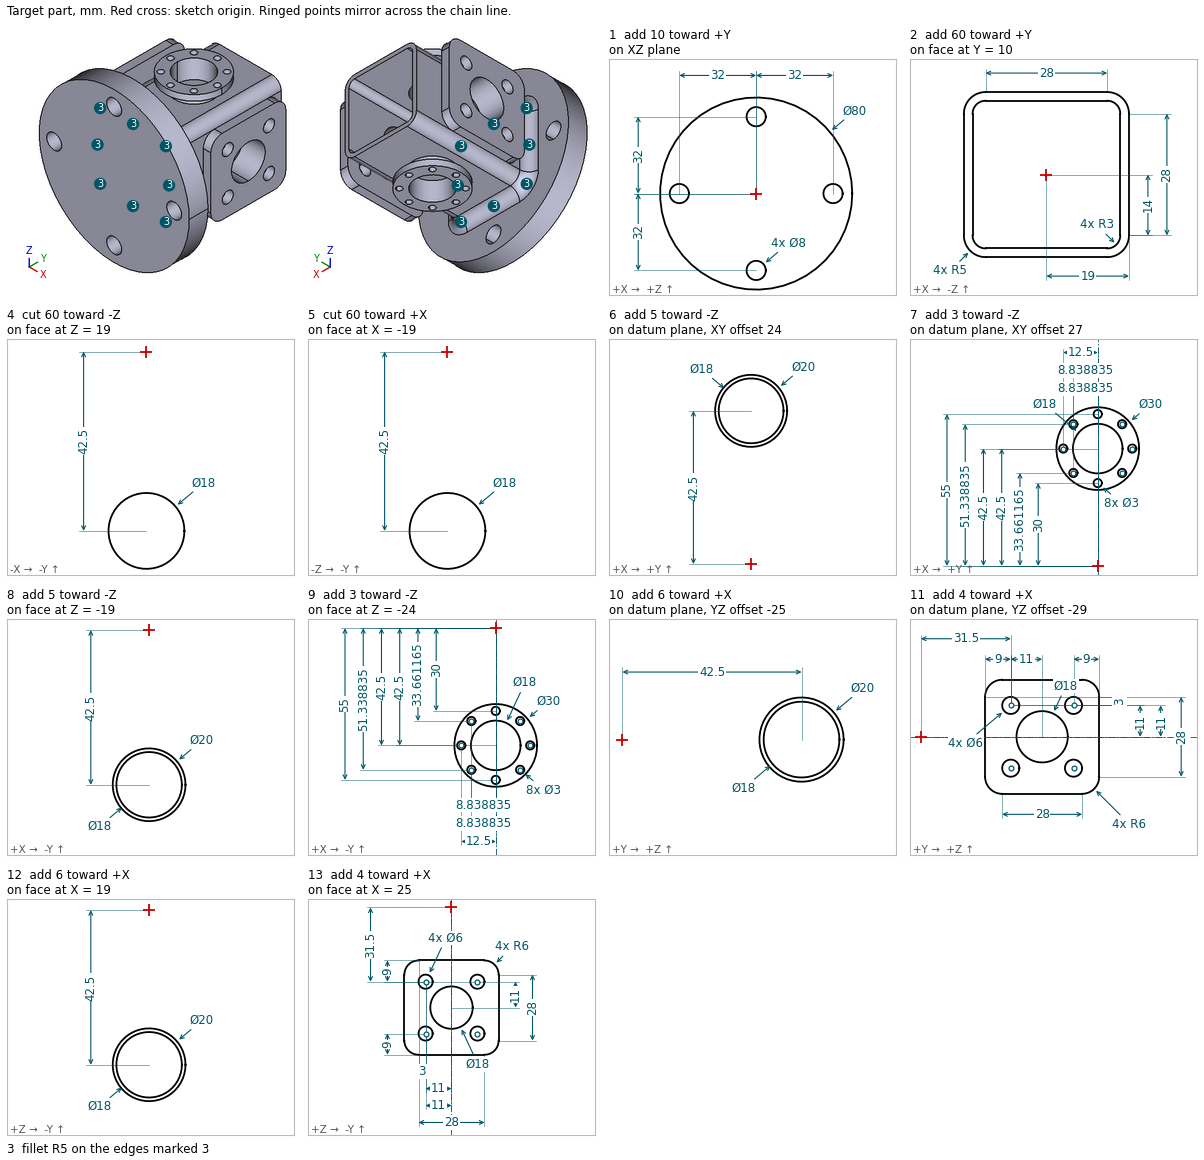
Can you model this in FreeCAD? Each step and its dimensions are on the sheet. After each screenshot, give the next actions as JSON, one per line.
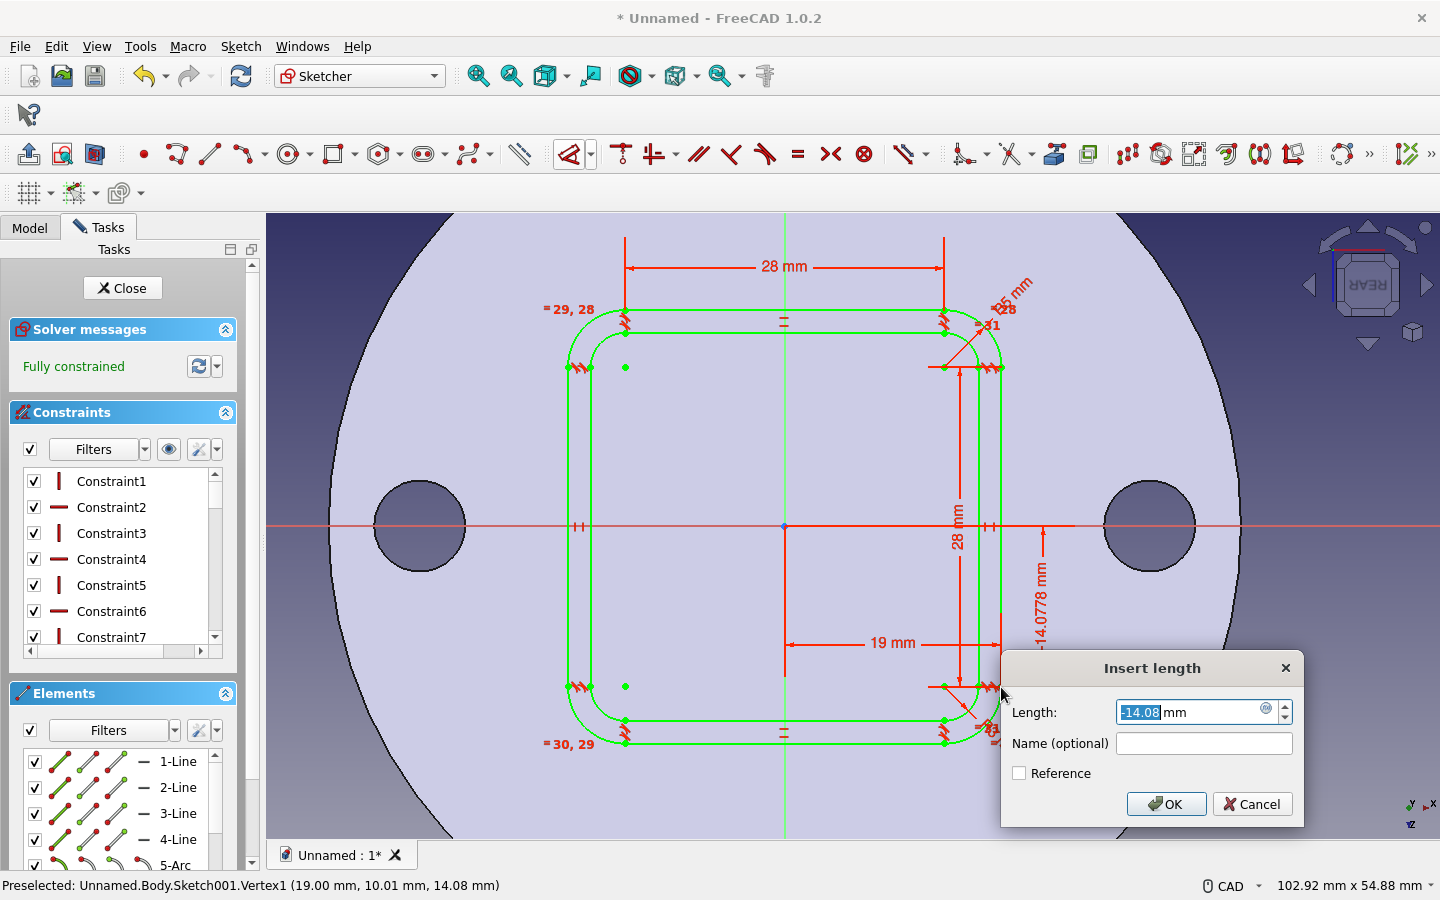
{"action": "type", "text": "-14"}
{"action": "key", "text": "Return"}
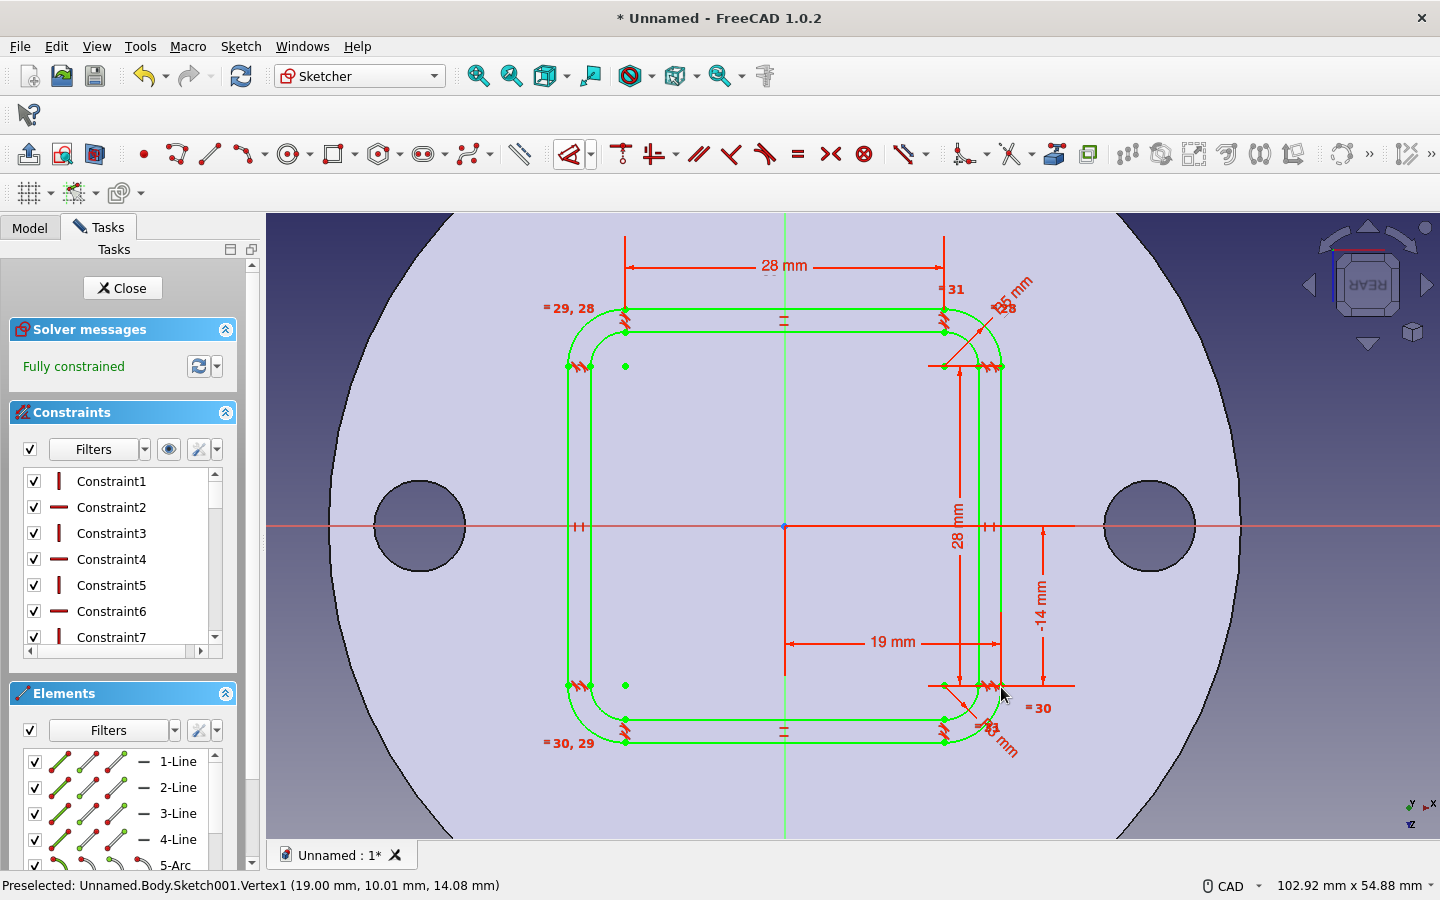
{"action": "left_click", "coordinate": [123, 288]}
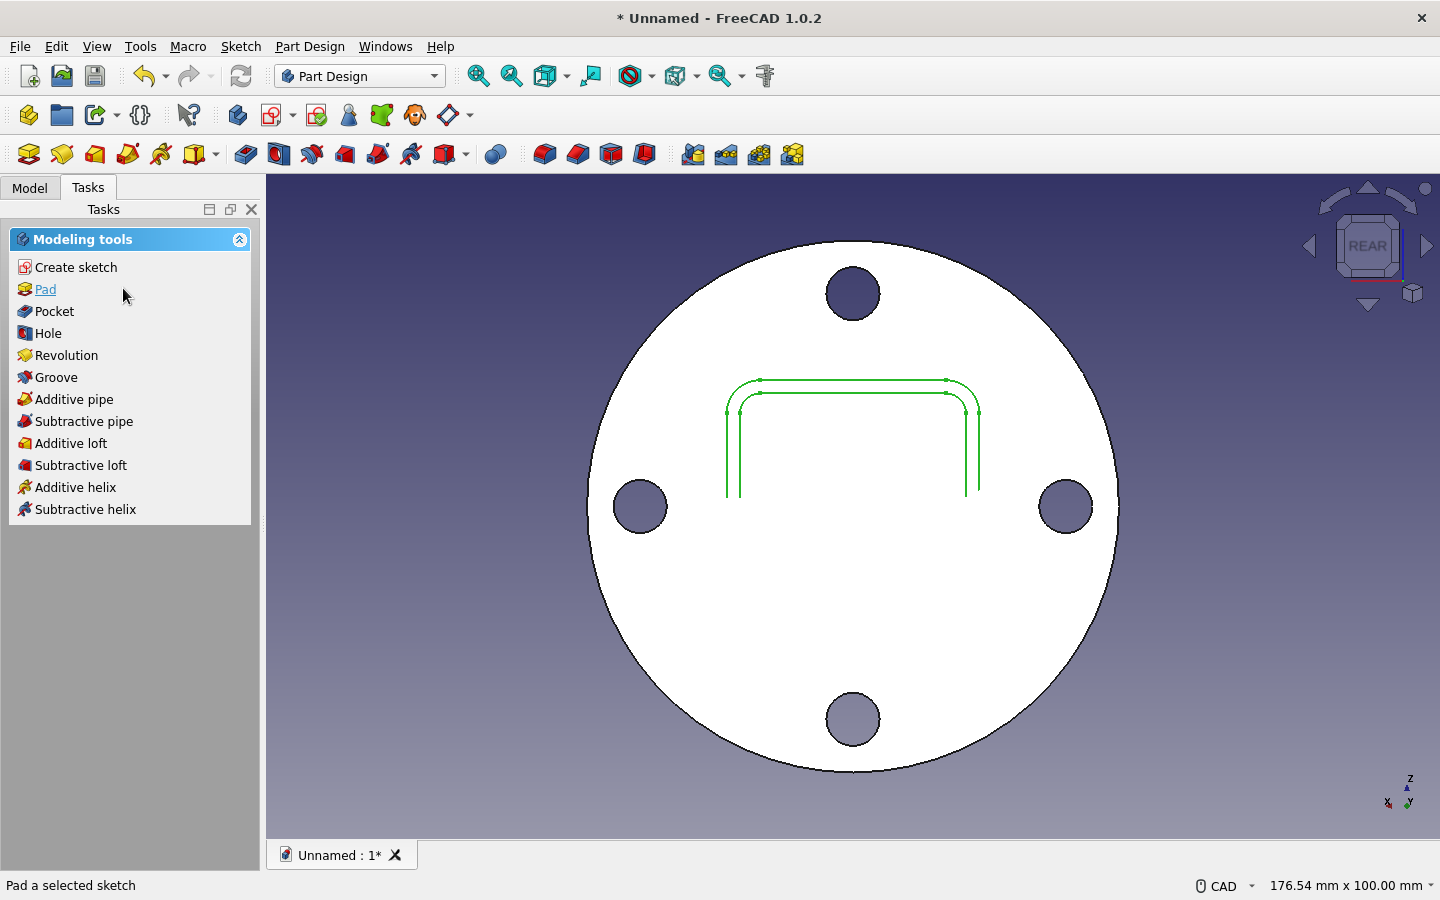
{"action": "left_click", "coordinate": [29, 154]}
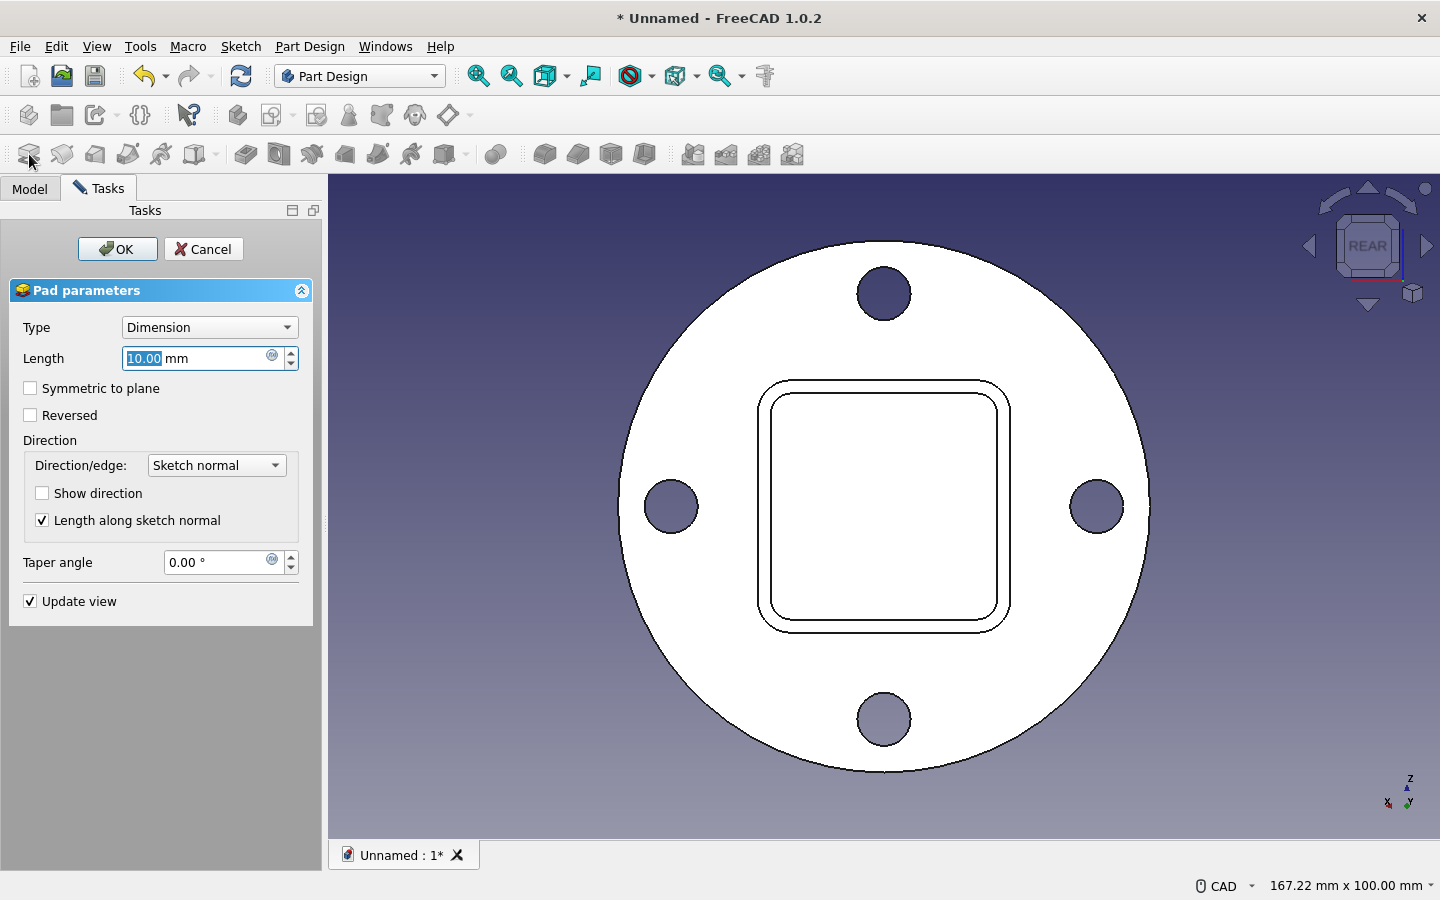
{"action": "type", "text": "60"}
{"action": "key", "text": "Tab"}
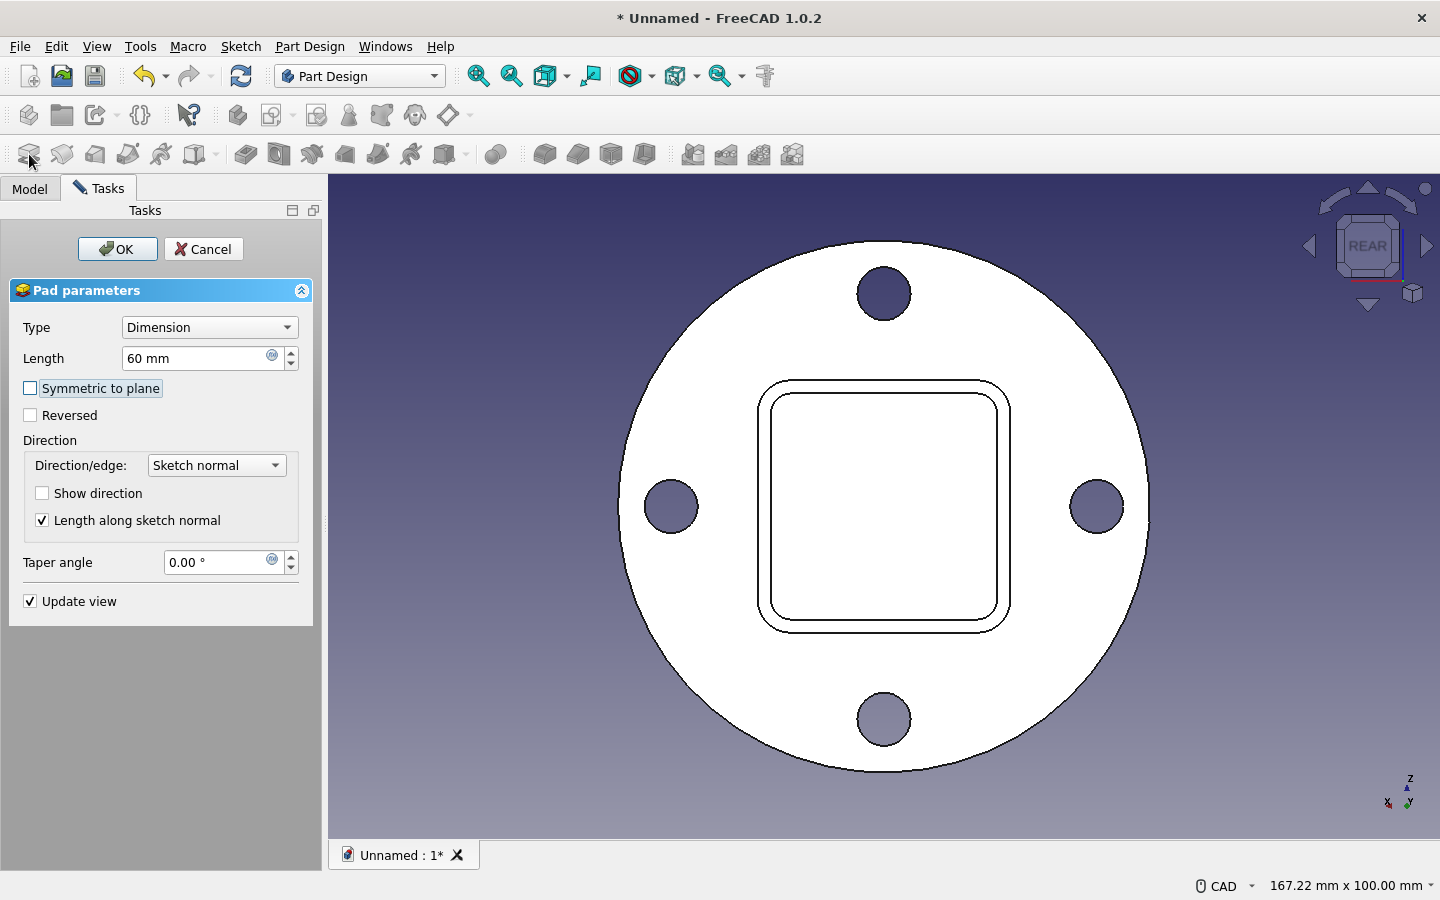
{"action": "left_click", "coordinate": [118, 249]}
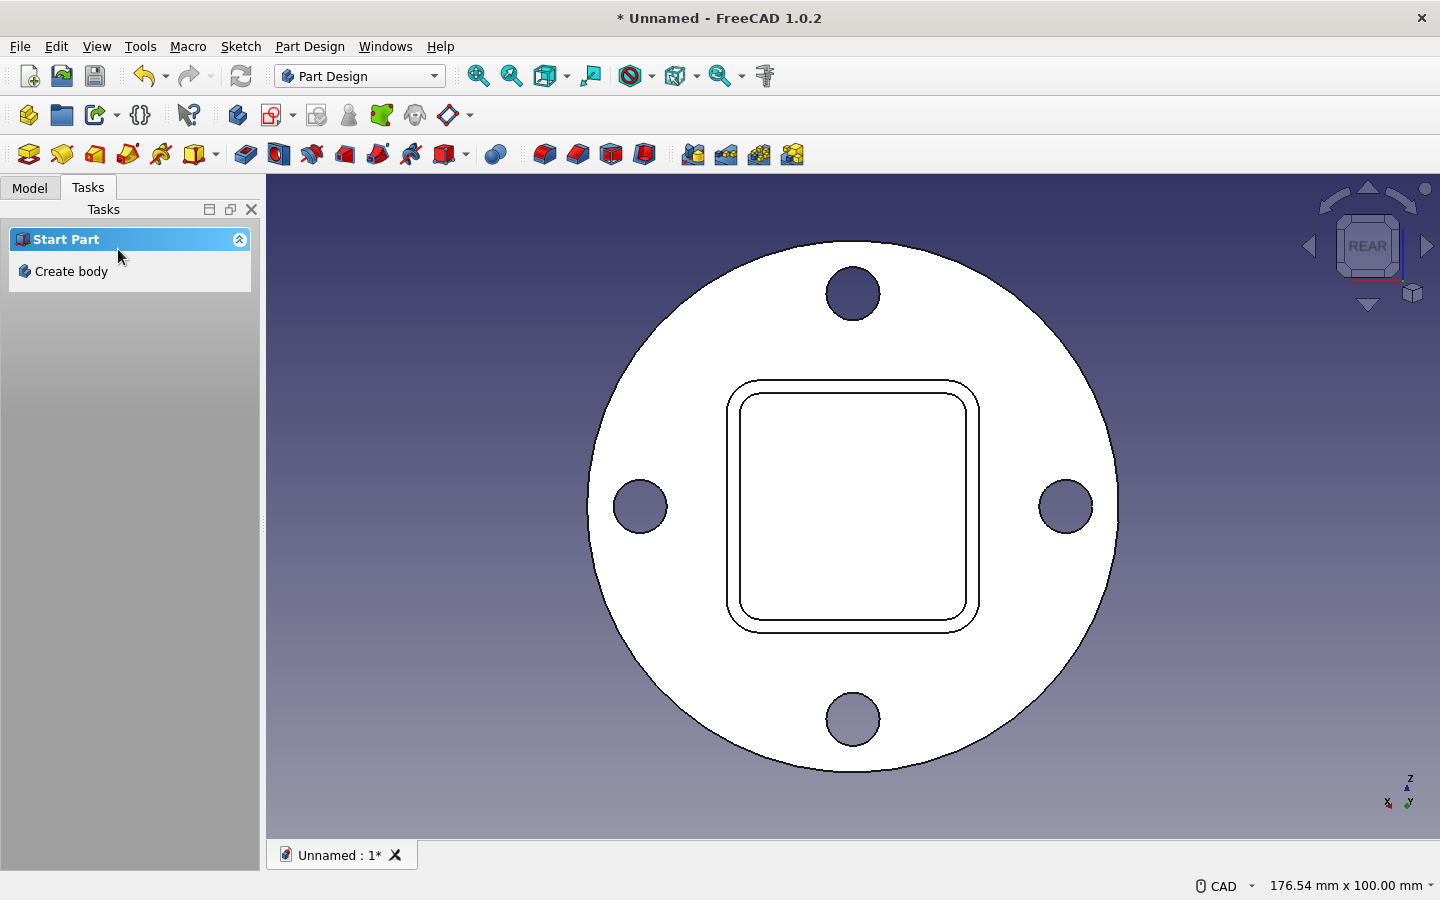
{"action": "key", "text": "0"}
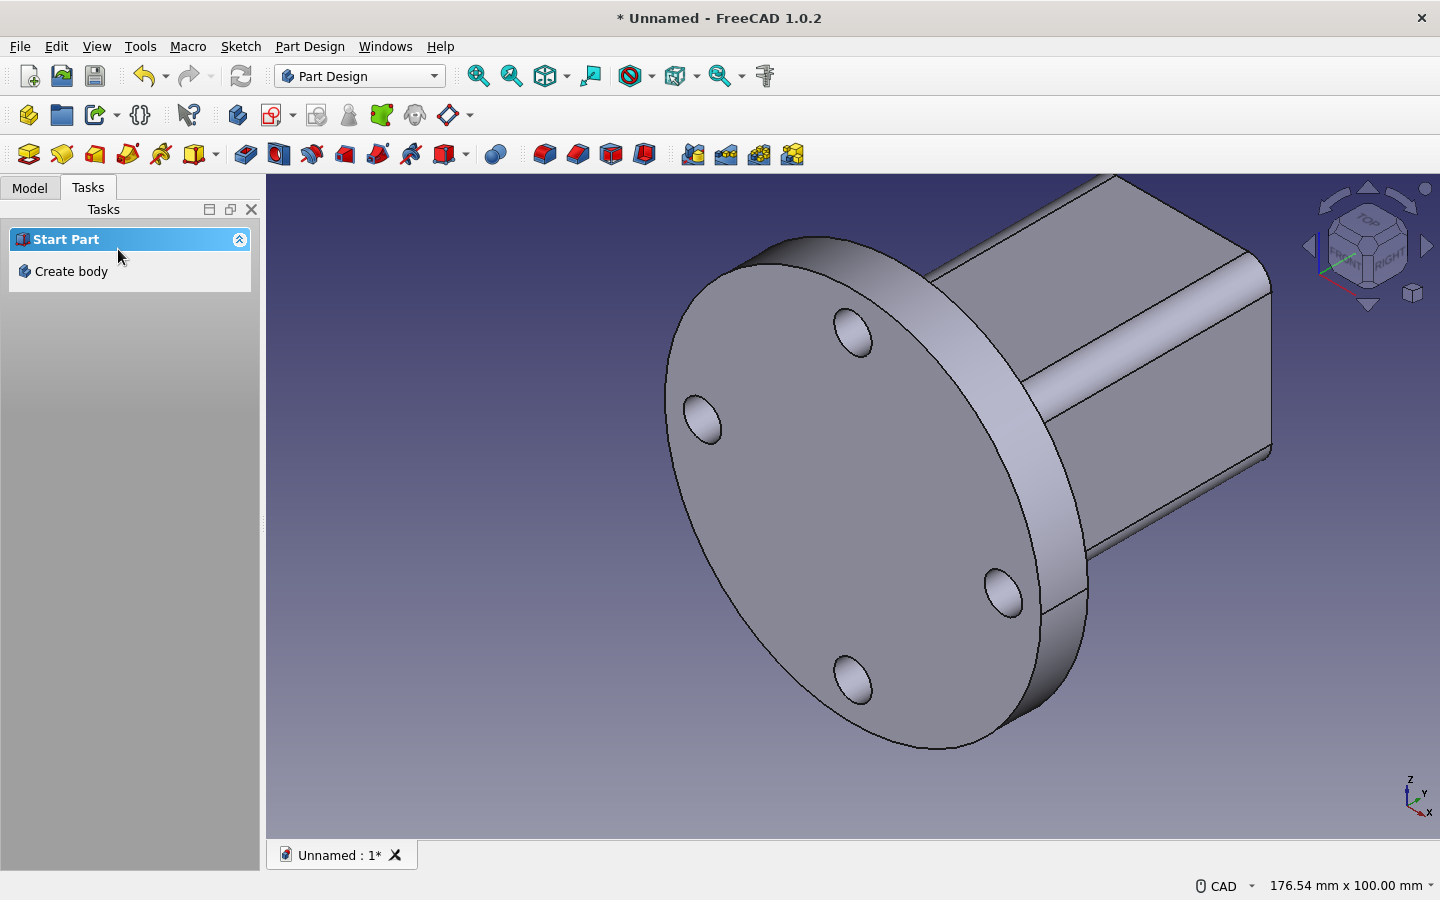
{"action": "key", "text": "v f"}